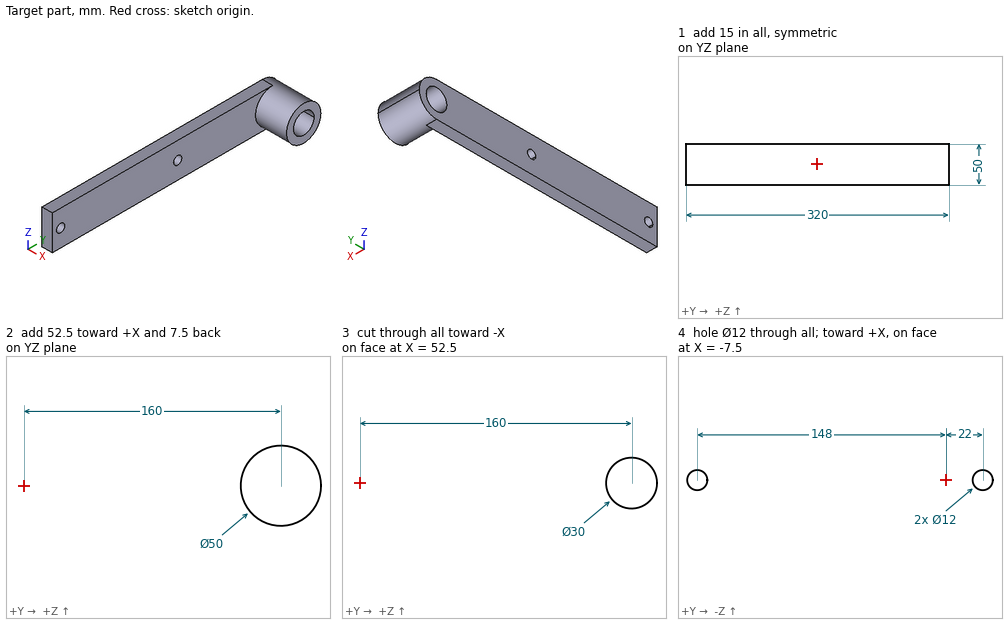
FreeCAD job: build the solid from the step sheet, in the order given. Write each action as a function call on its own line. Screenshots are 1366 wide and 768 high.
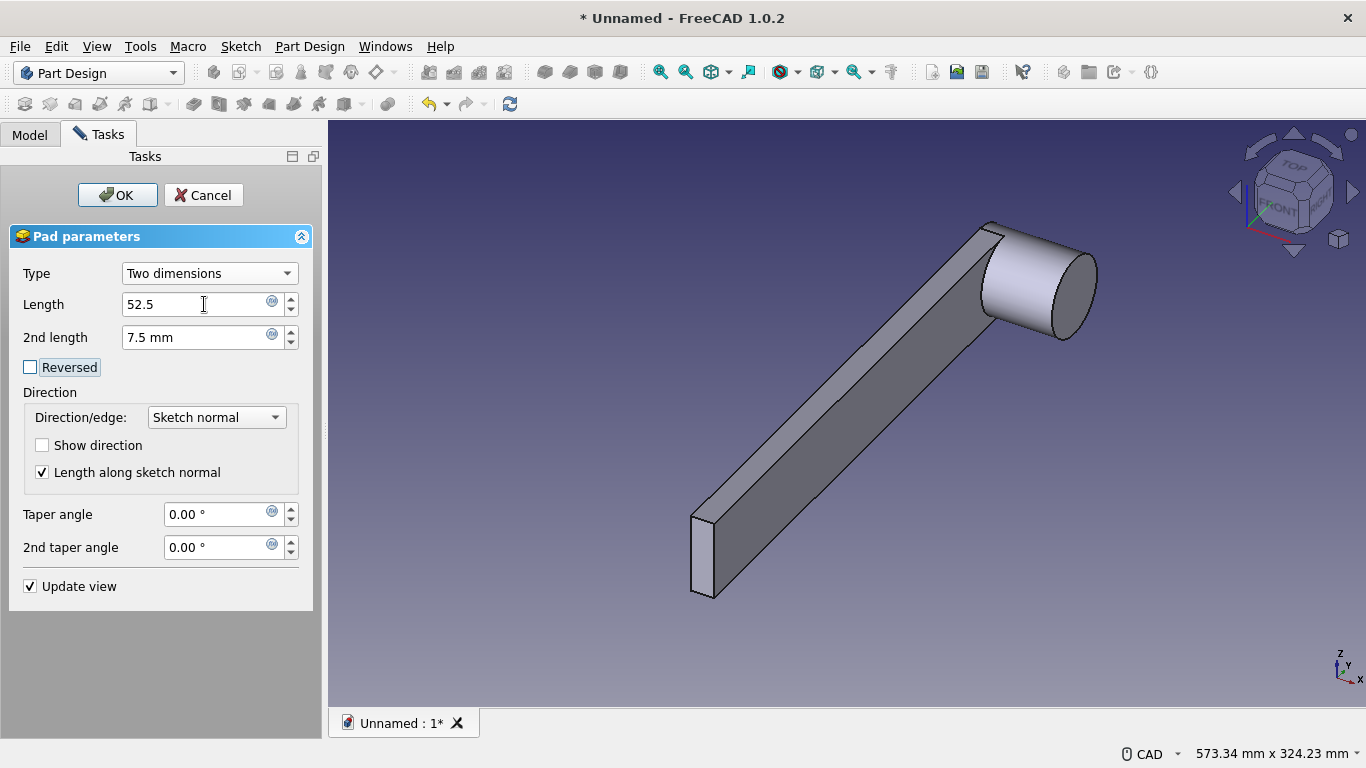
click(118, 195)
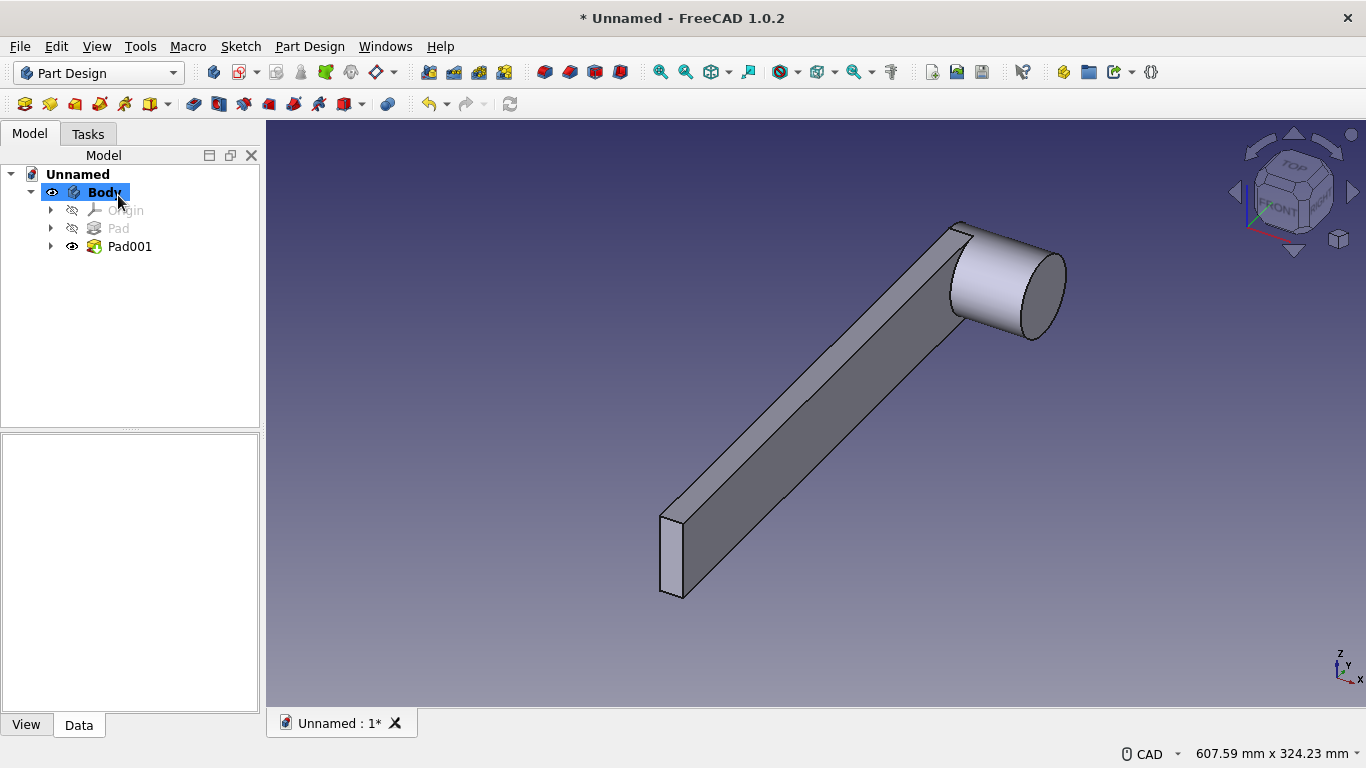
click(1043, 296)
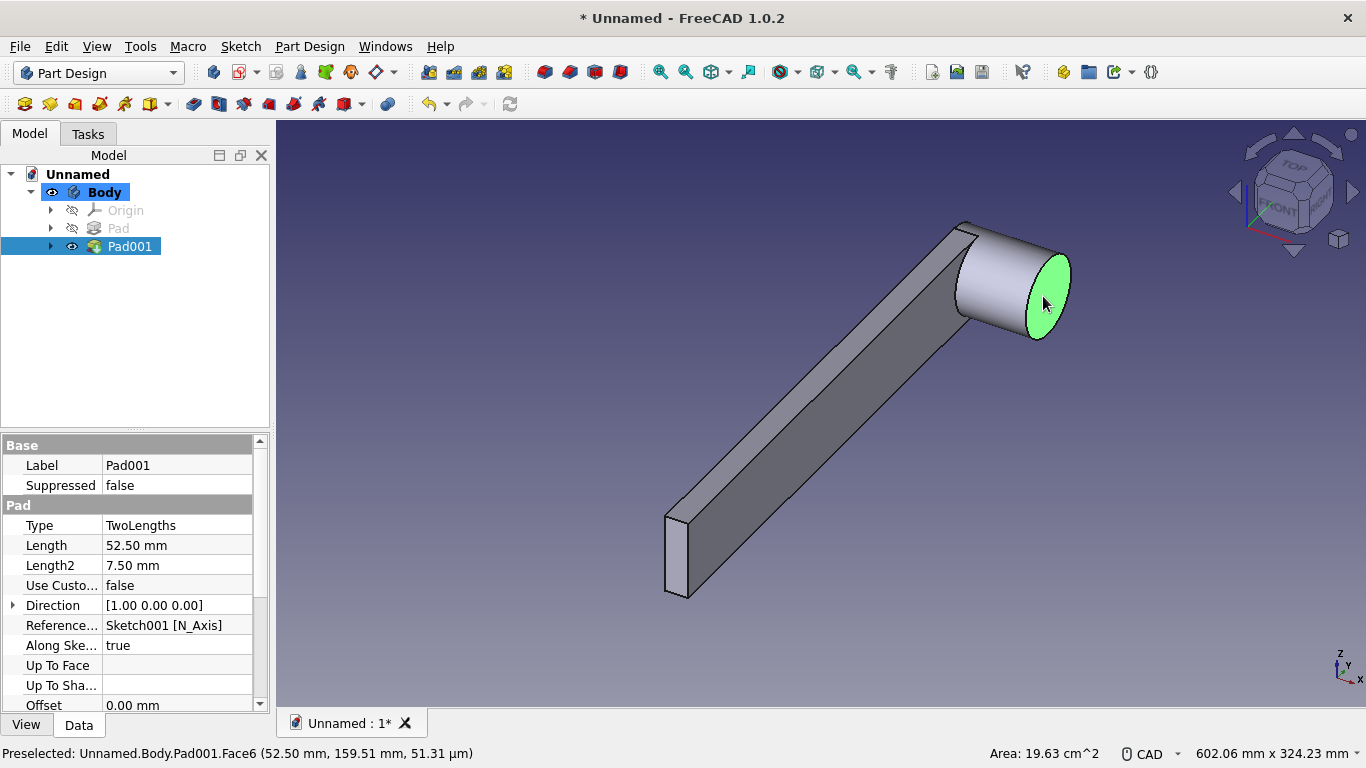
click(238, 72)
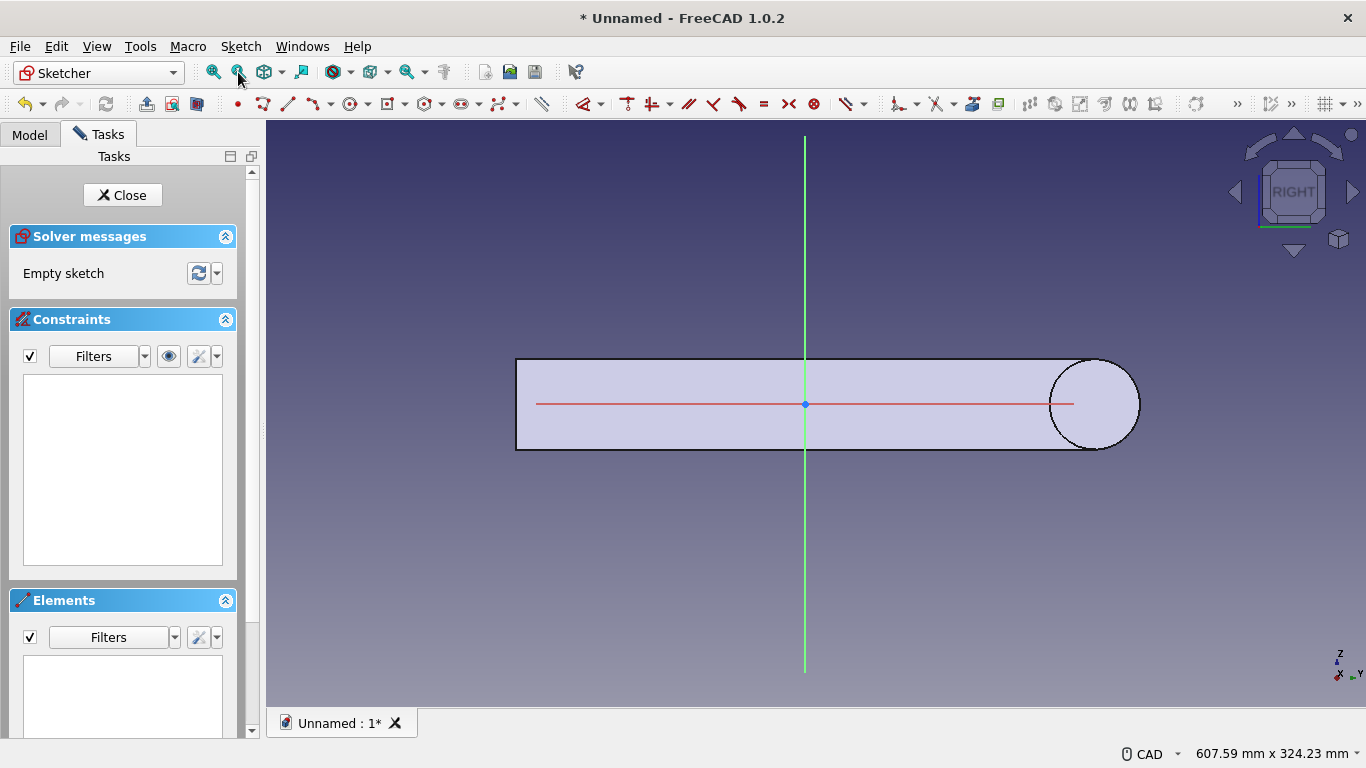
scroll(1149, 403, up, 10)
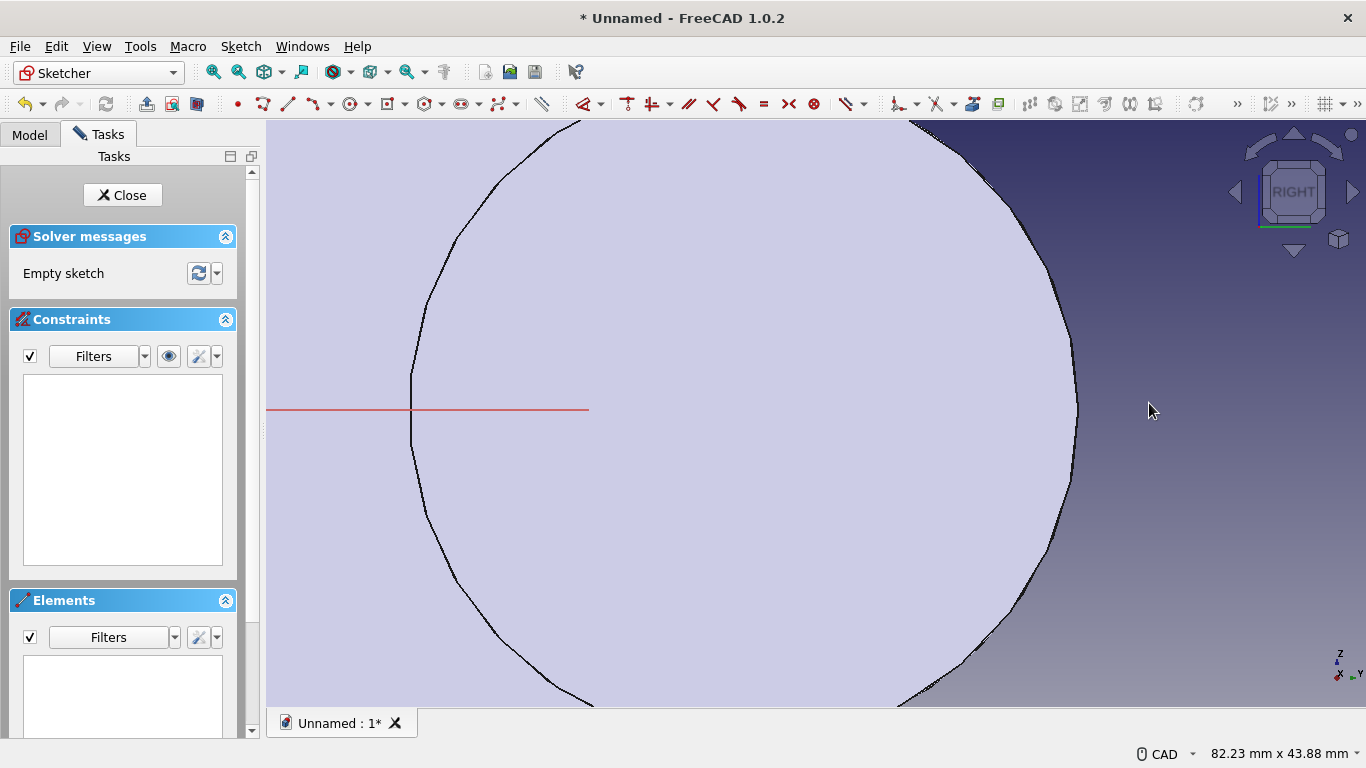
click(350, 104)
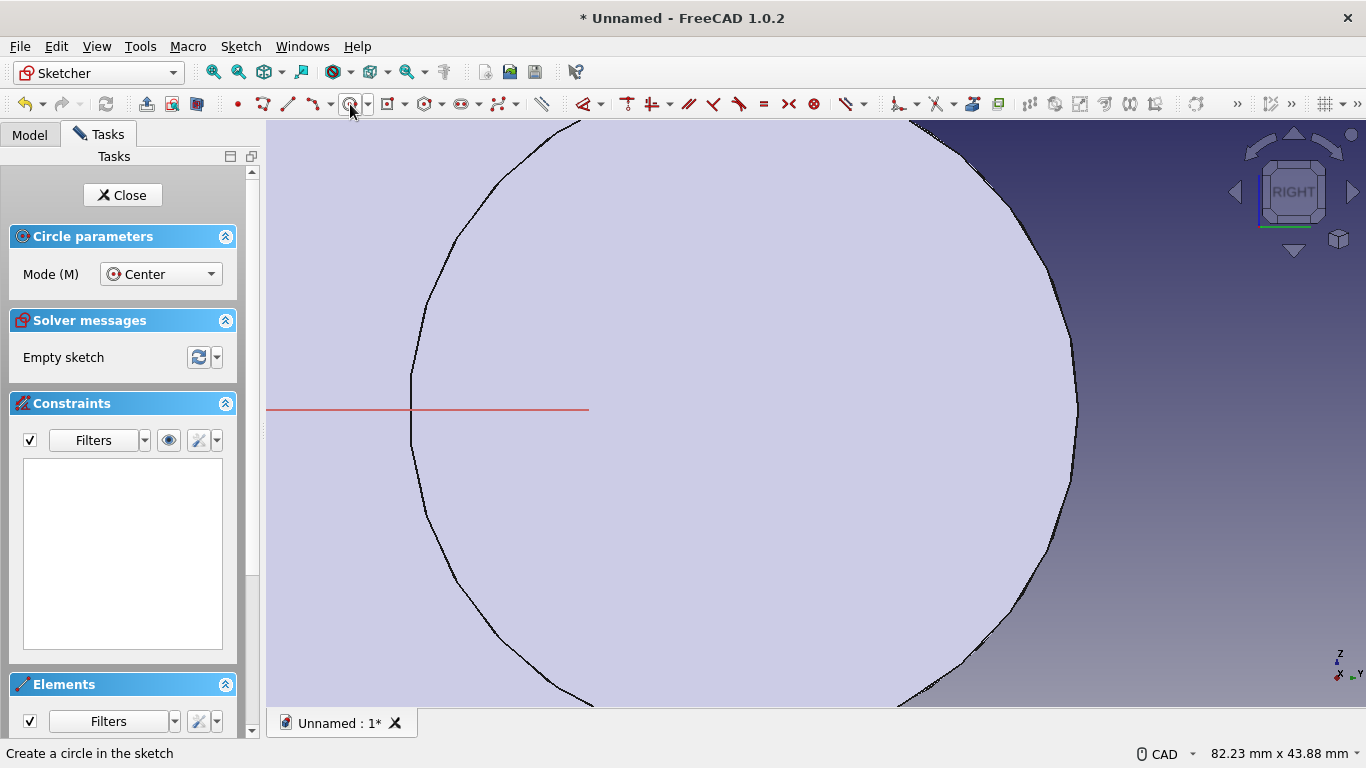
click(744, 410)
click(886, 268)
key(Escape)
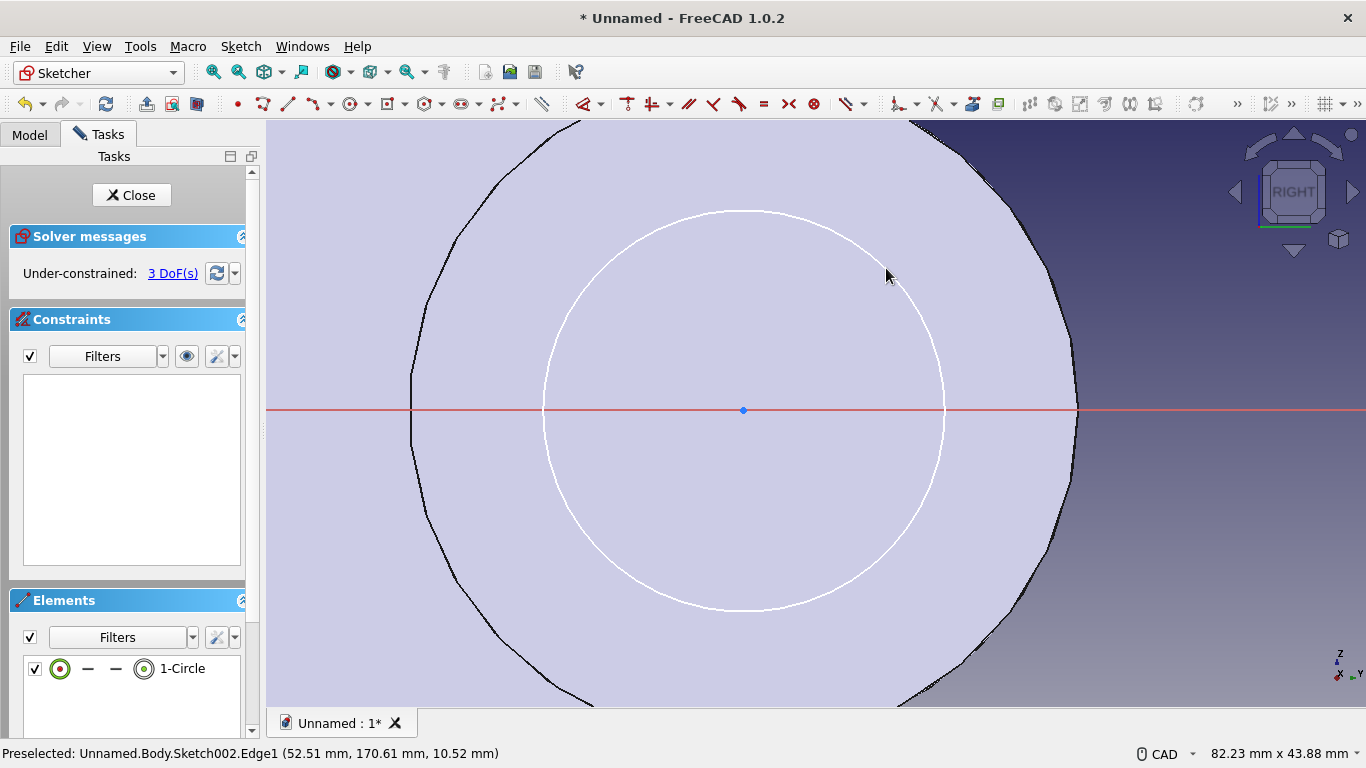
click(744, 411)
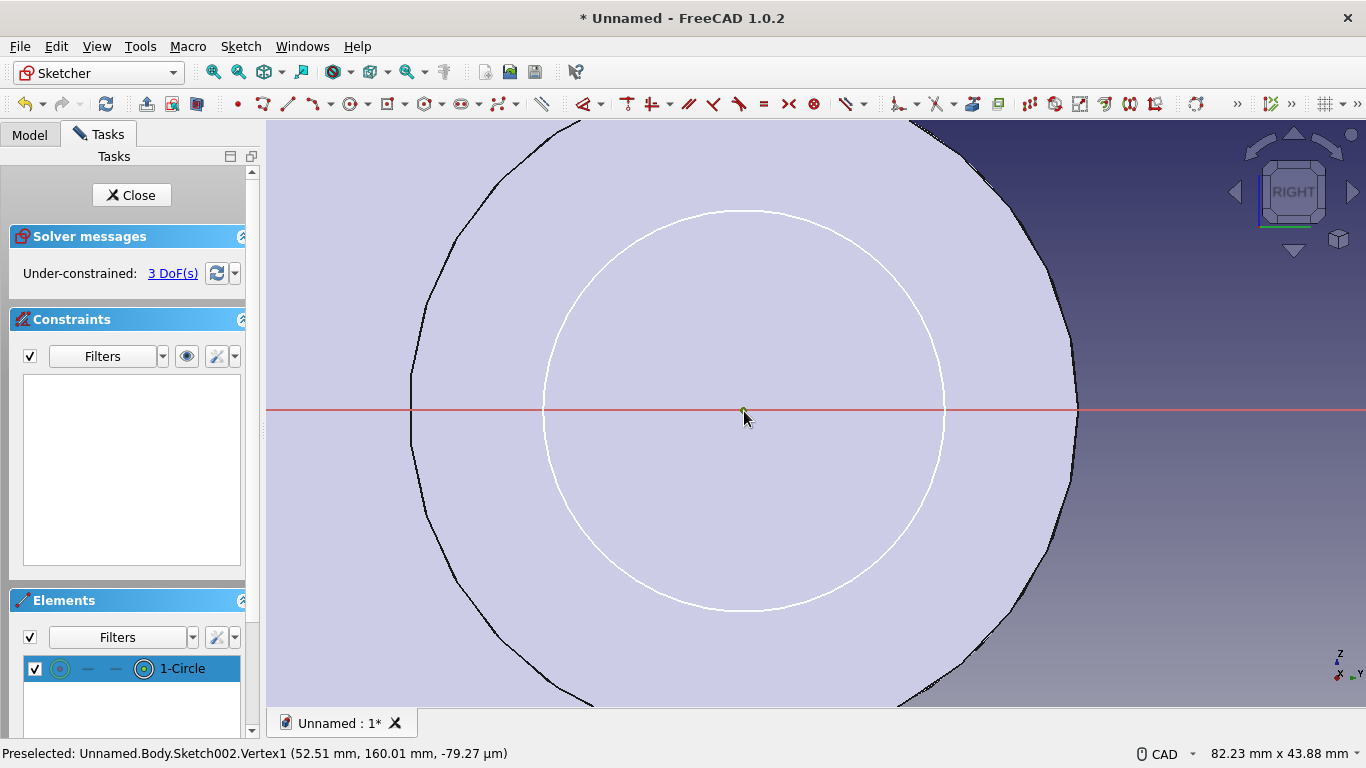
click(359, 410)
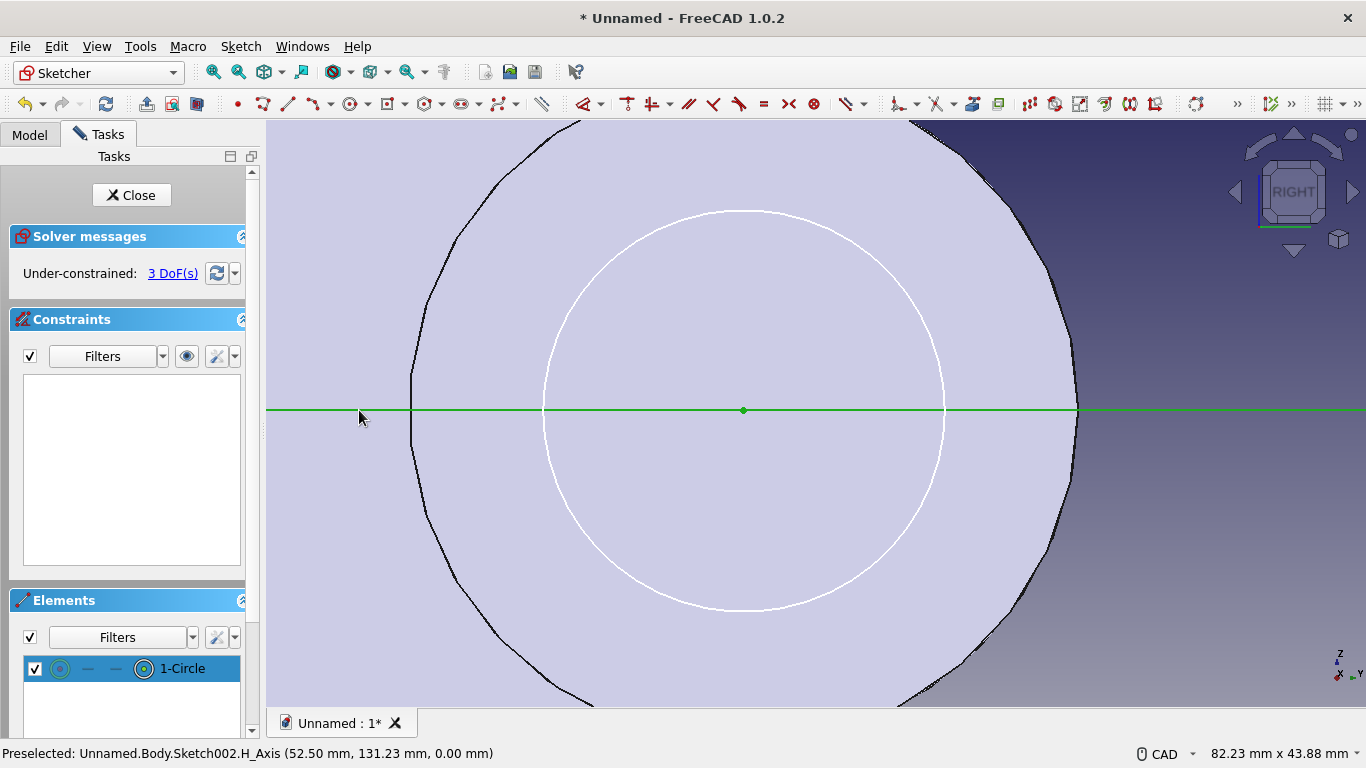
click(627, 104)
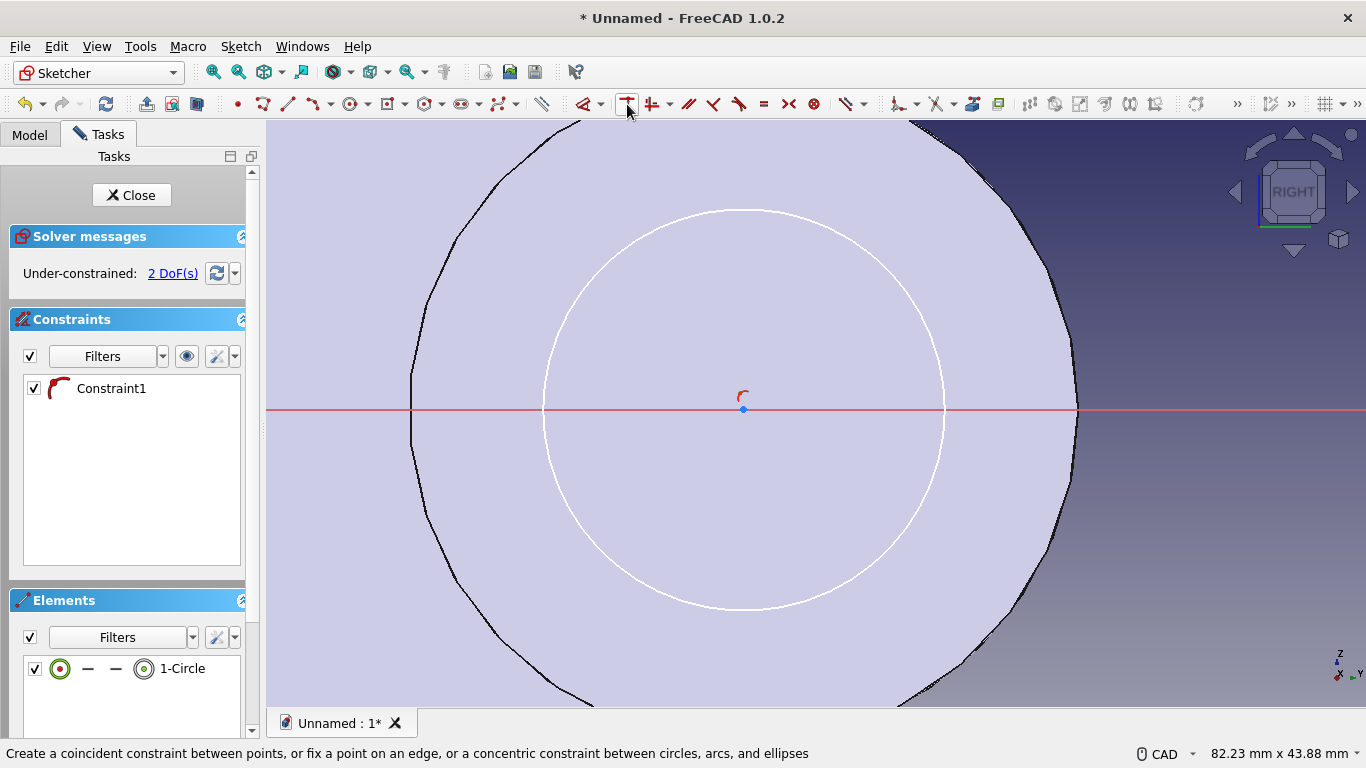
click(582, 104)